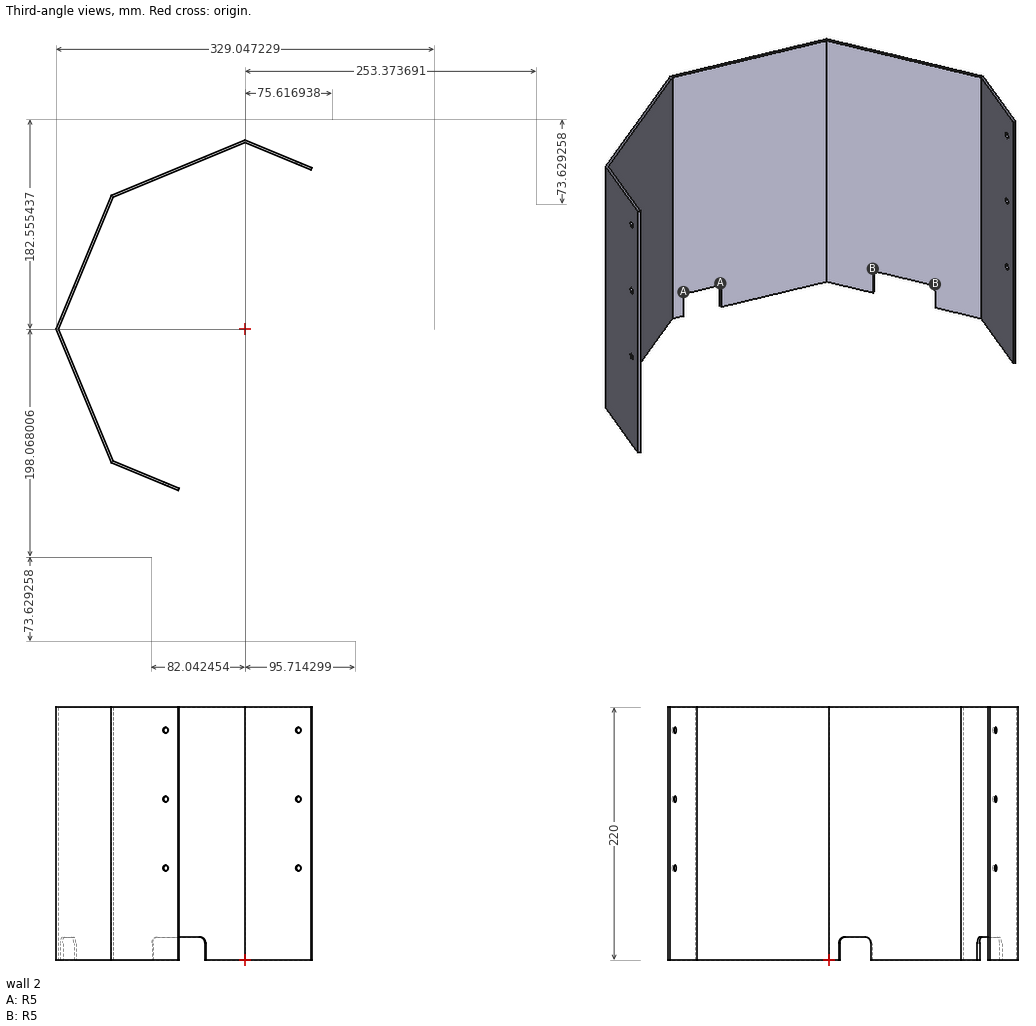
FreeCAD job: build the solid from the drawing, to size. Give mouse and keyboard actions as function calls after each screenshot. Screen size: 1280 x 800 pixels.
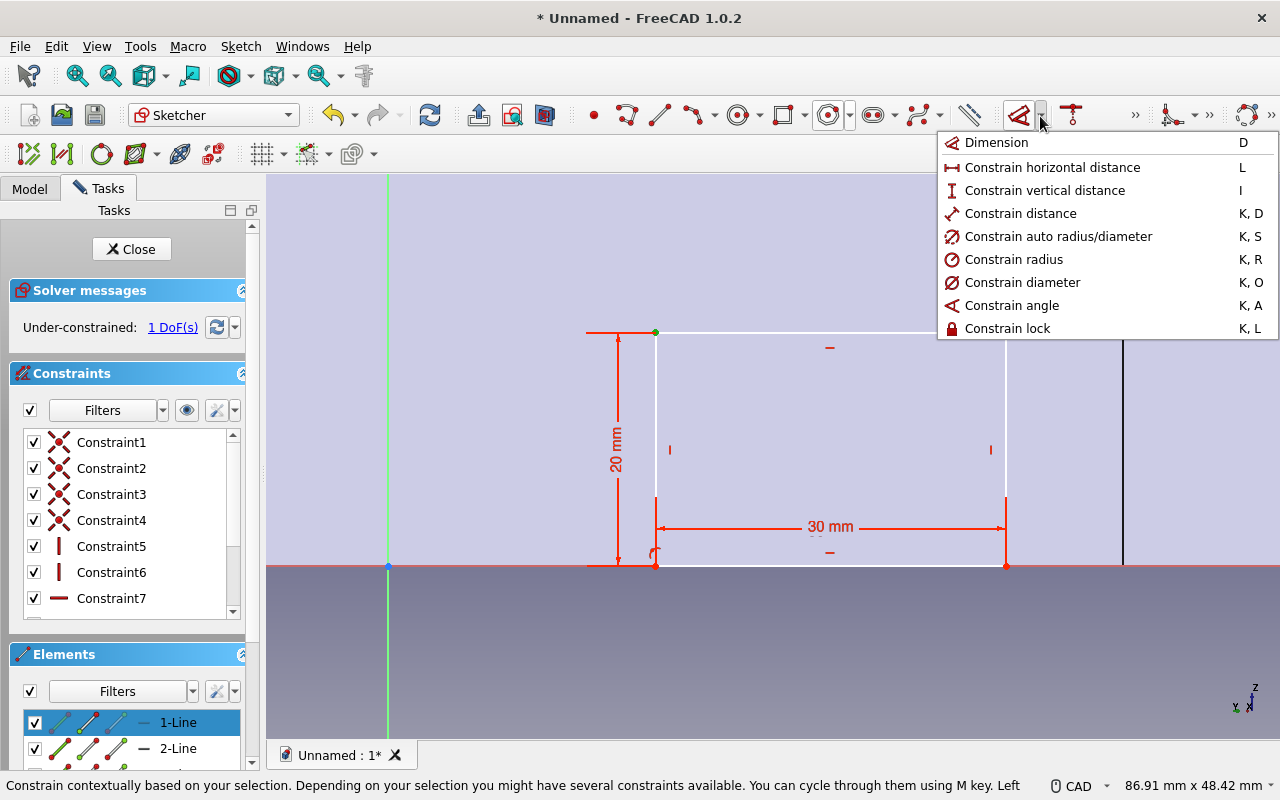
click(1108, 168)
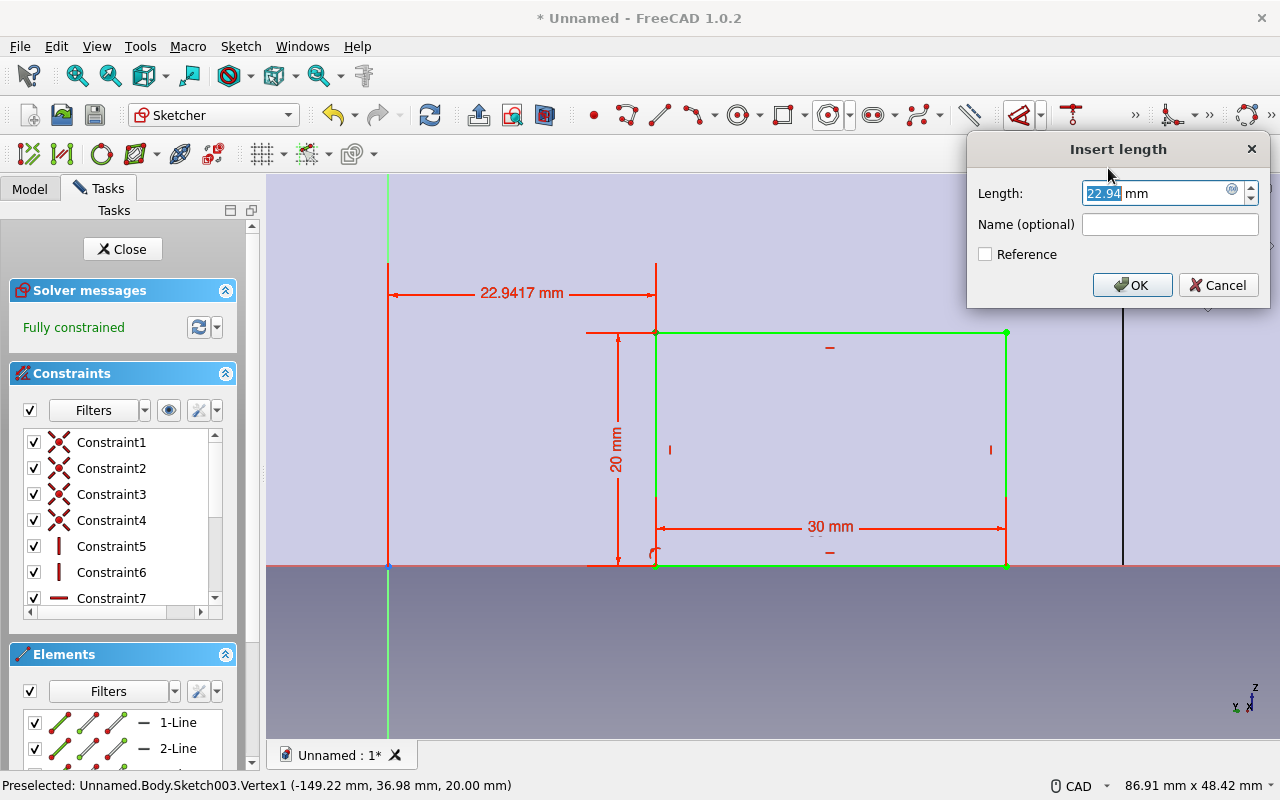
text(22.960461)
key(Return)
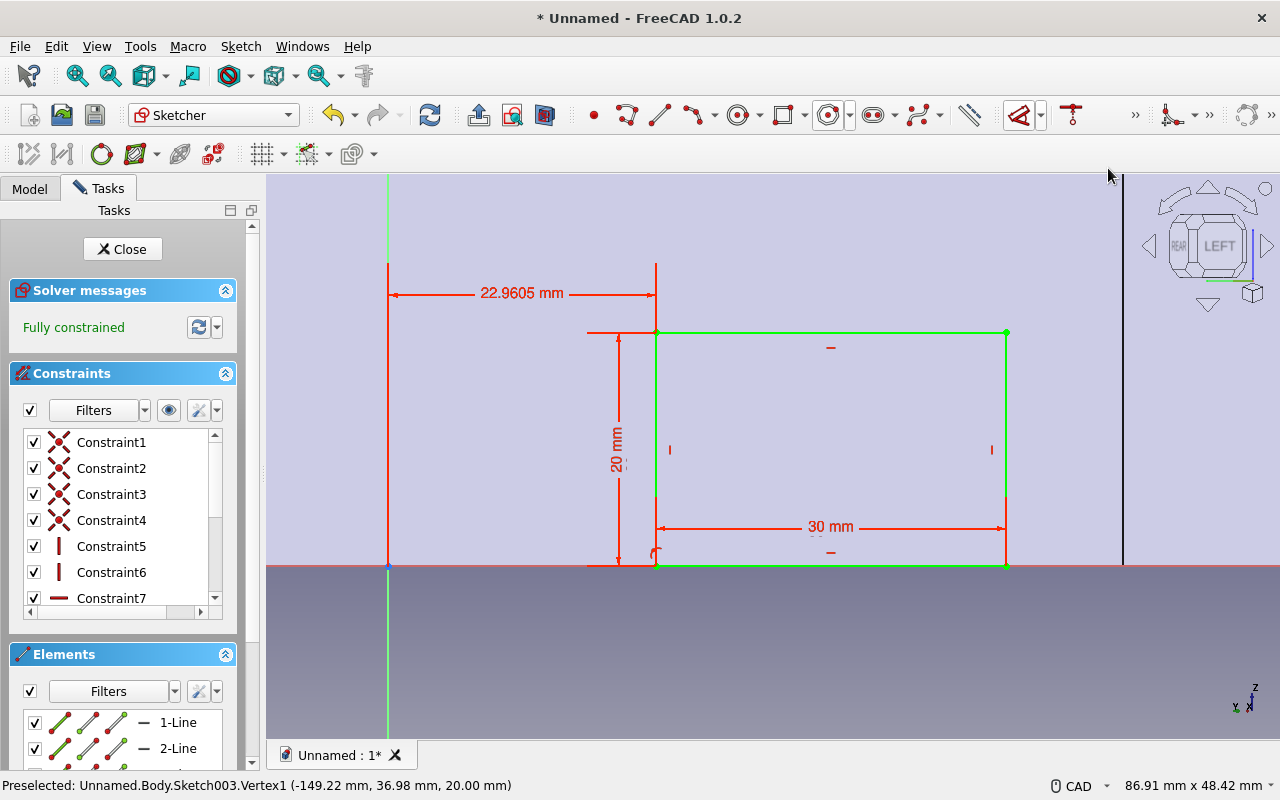
click(123, 249)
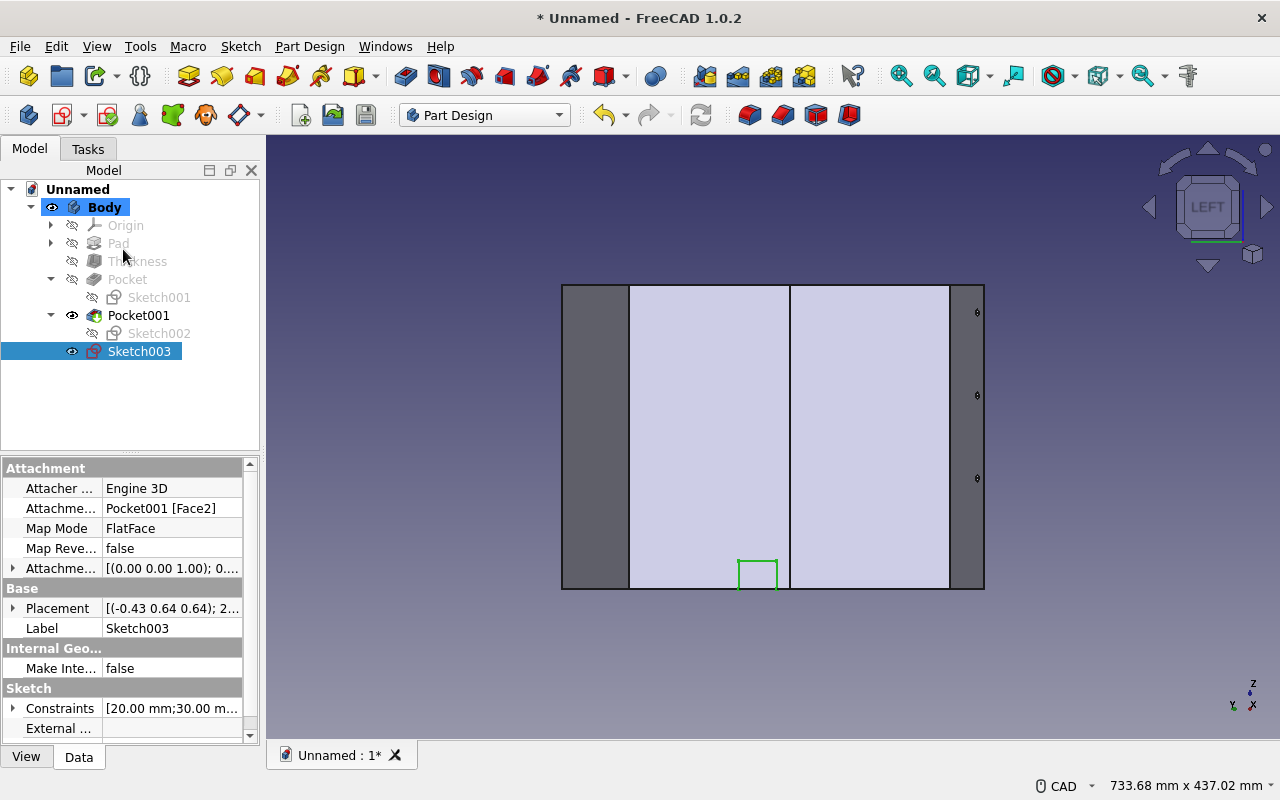
click(406, 76)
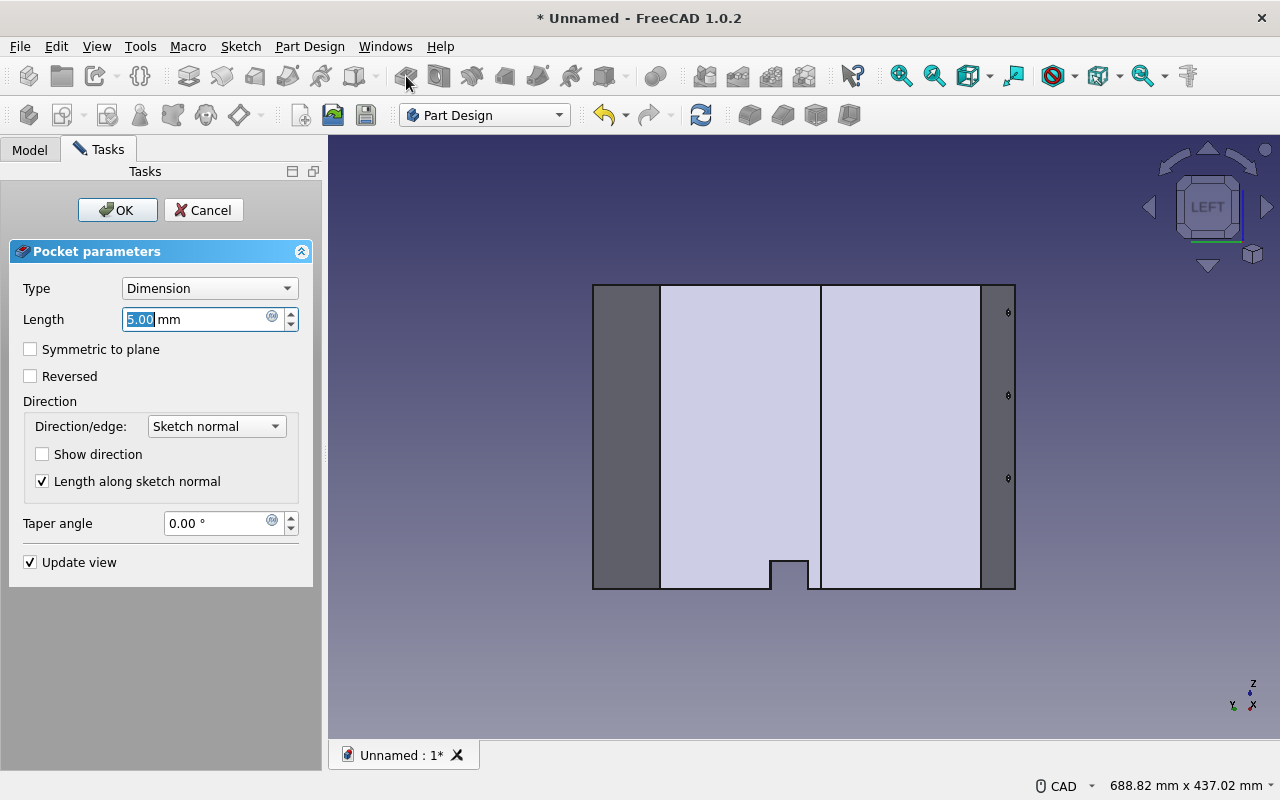
click(210, 288)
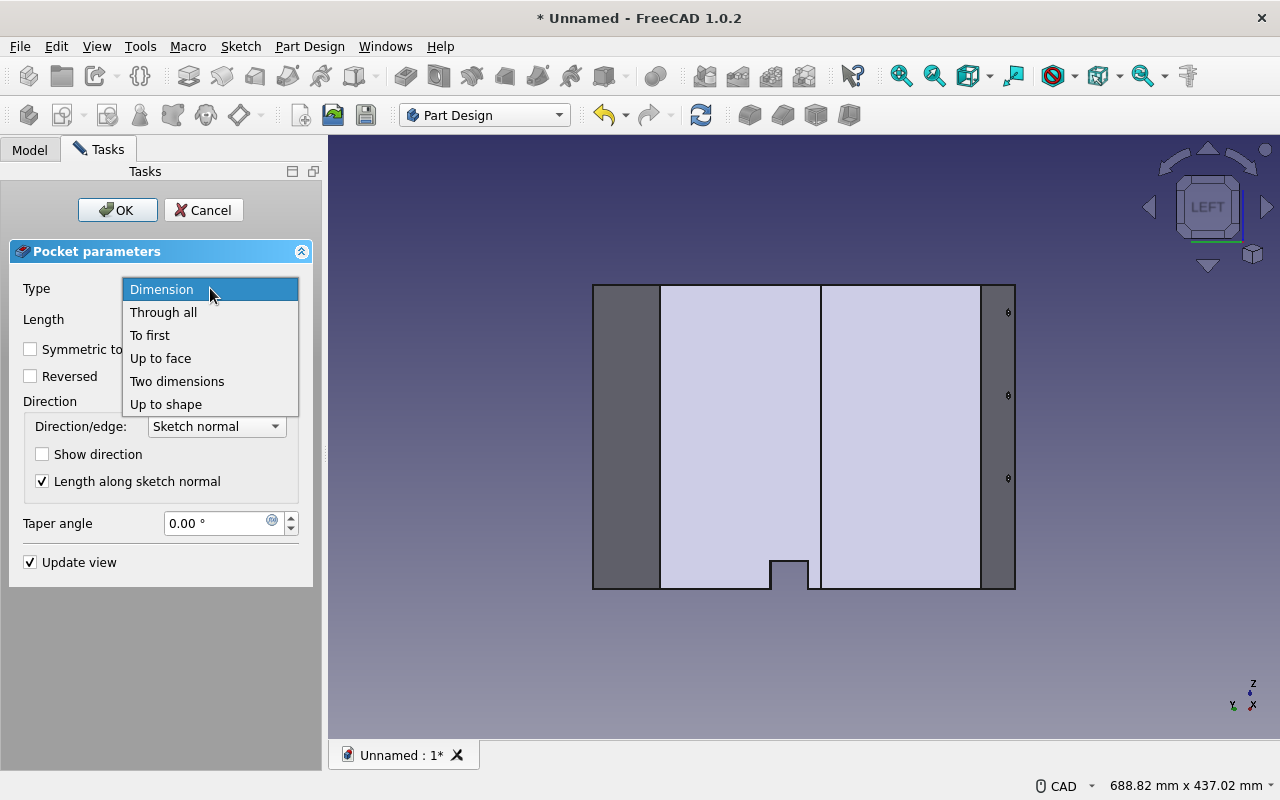
click(208, 312)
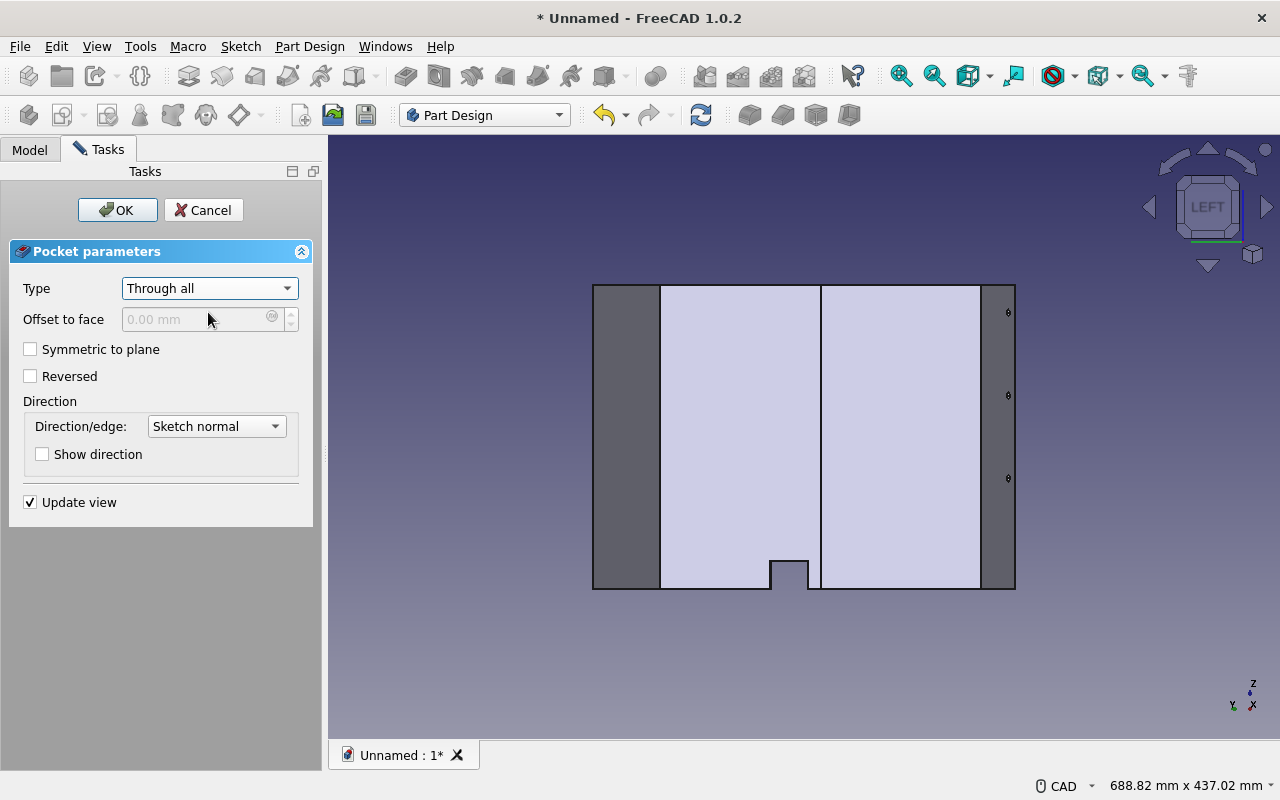
click(118, 210)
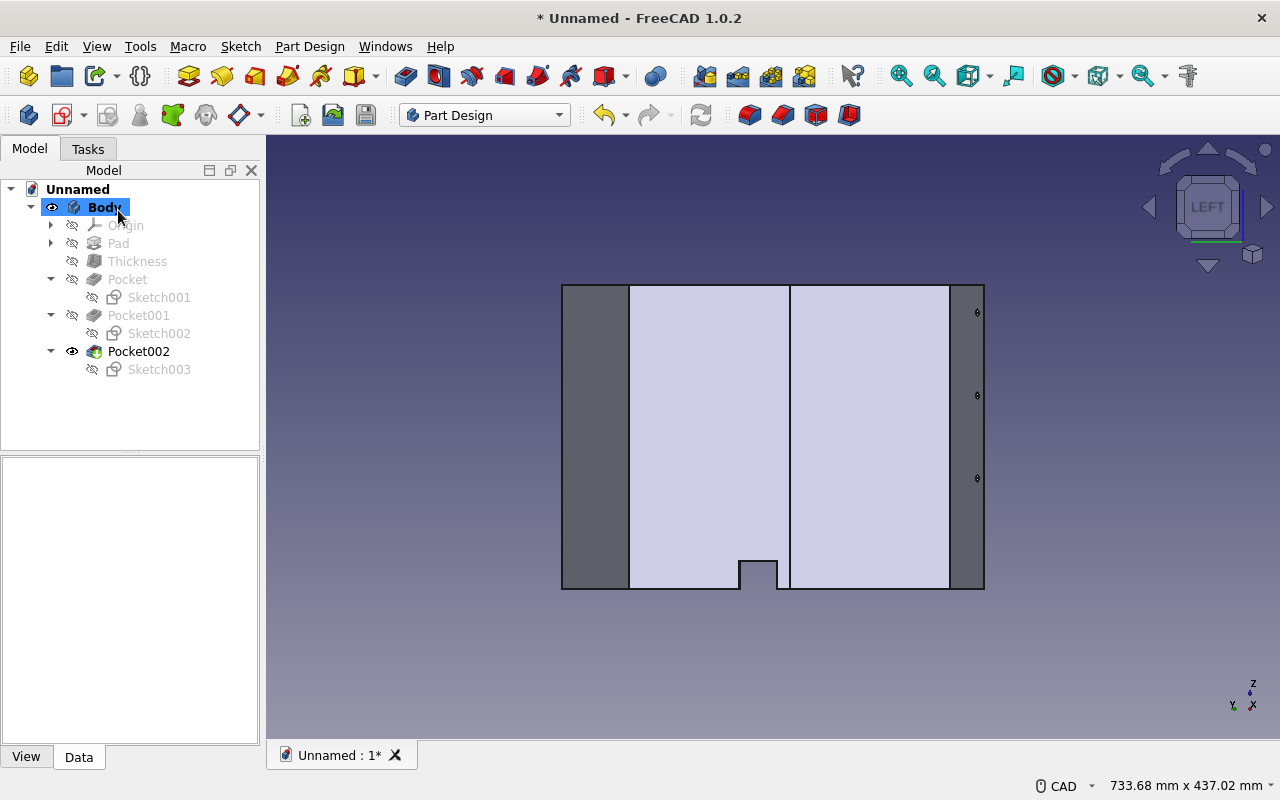
scroll(739, 560, up, 14)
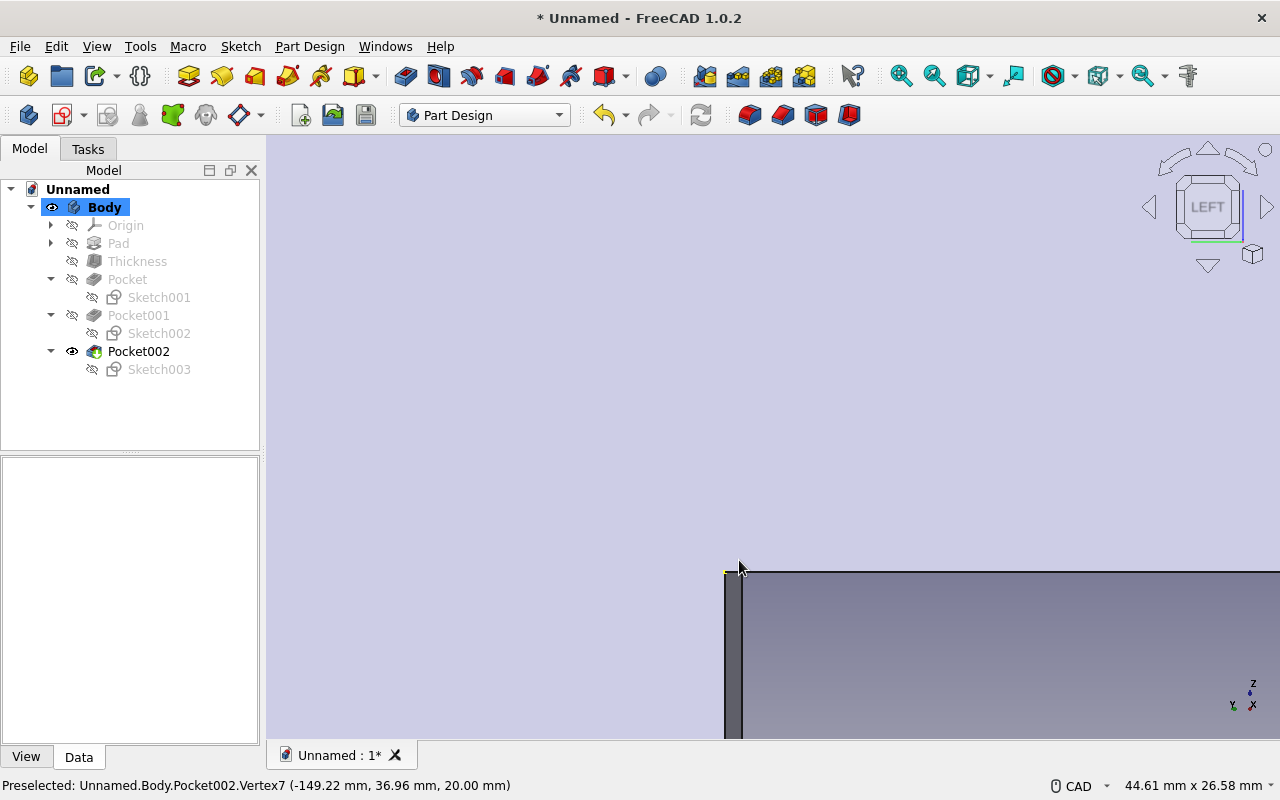
click(902, 76)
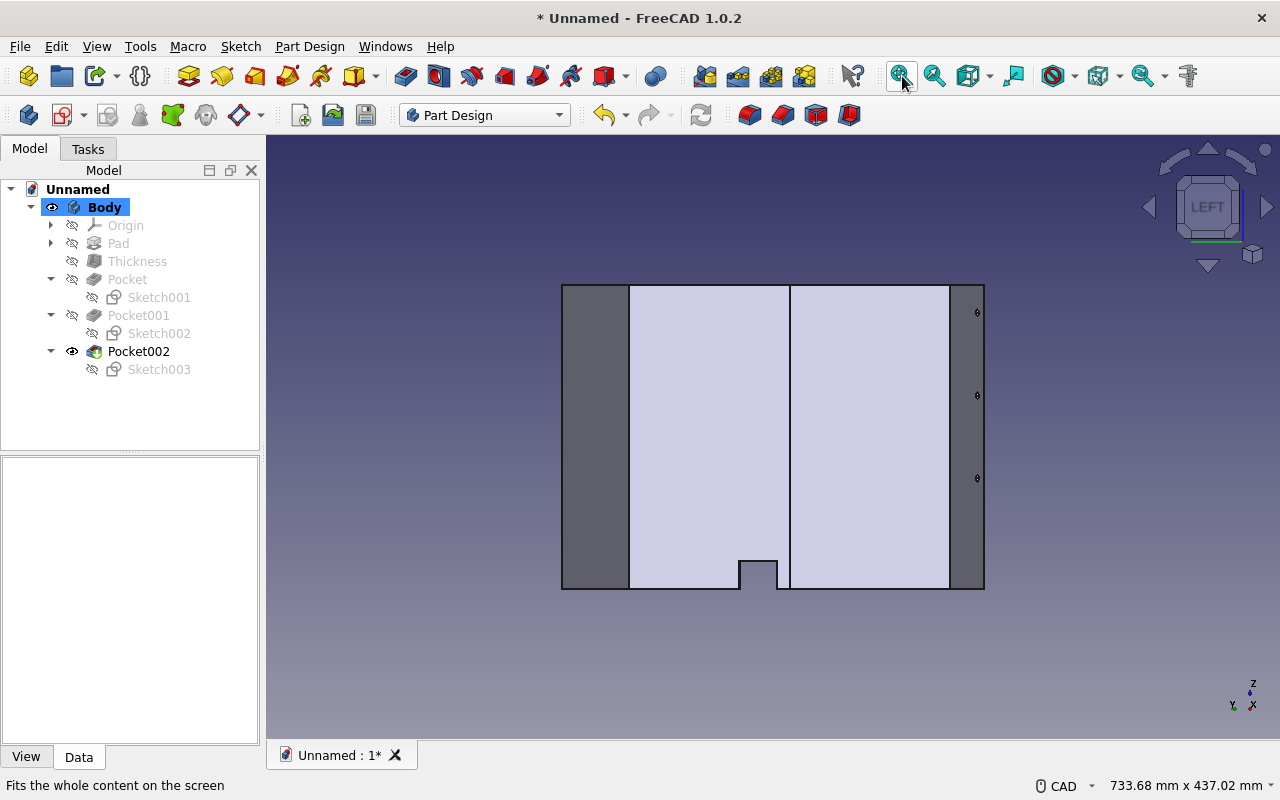
key(0)